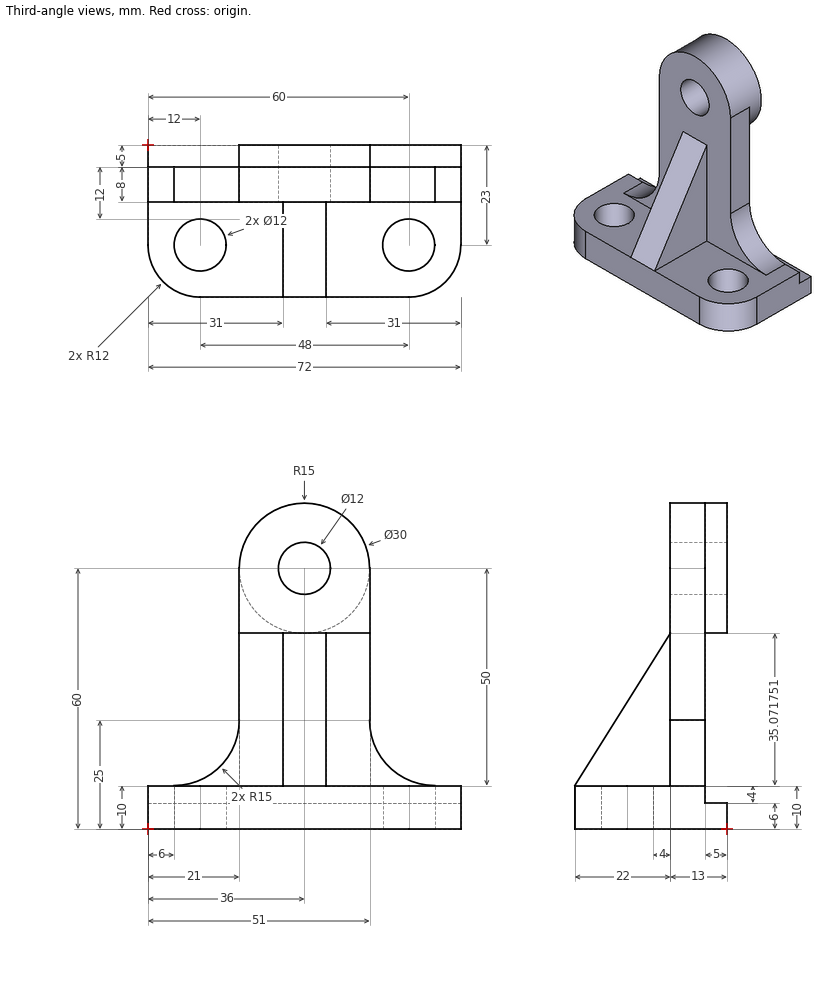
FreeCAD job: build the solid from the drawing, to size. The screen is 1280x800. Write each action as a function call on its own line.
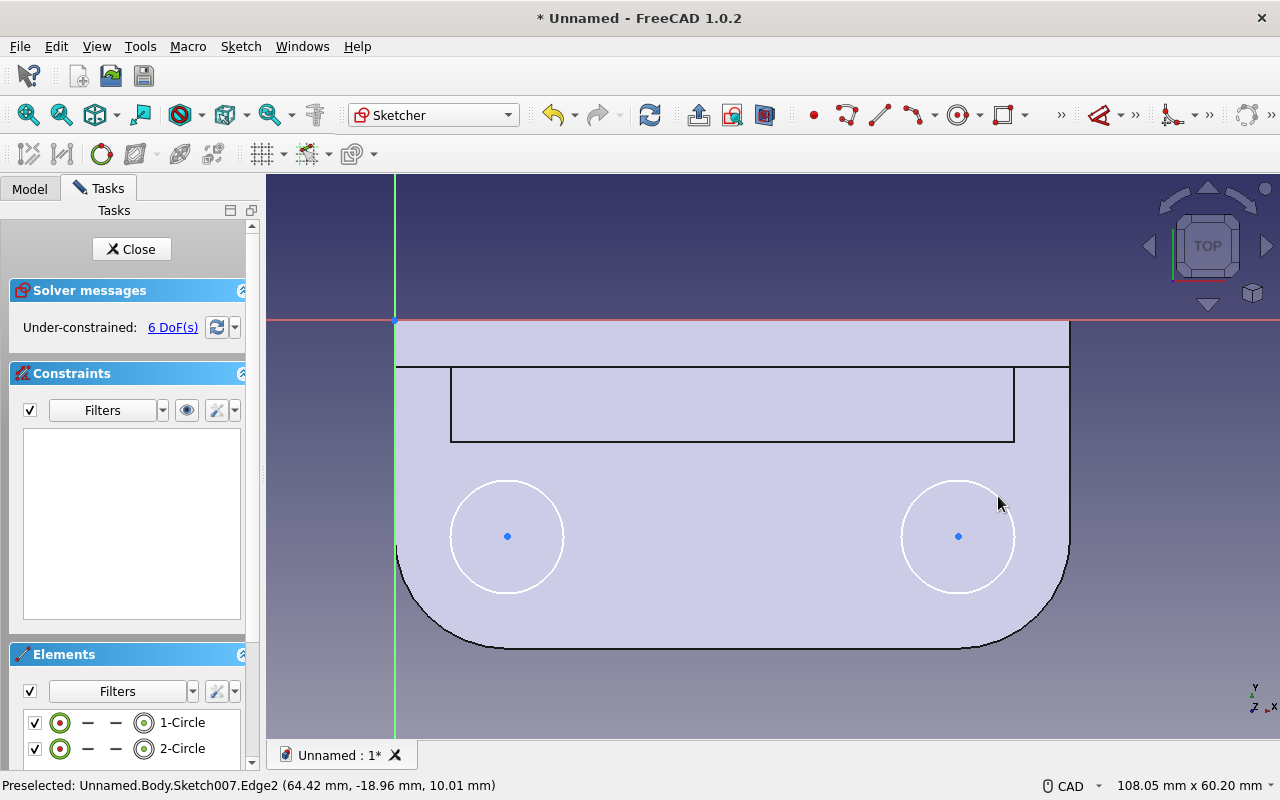
click(547, 497)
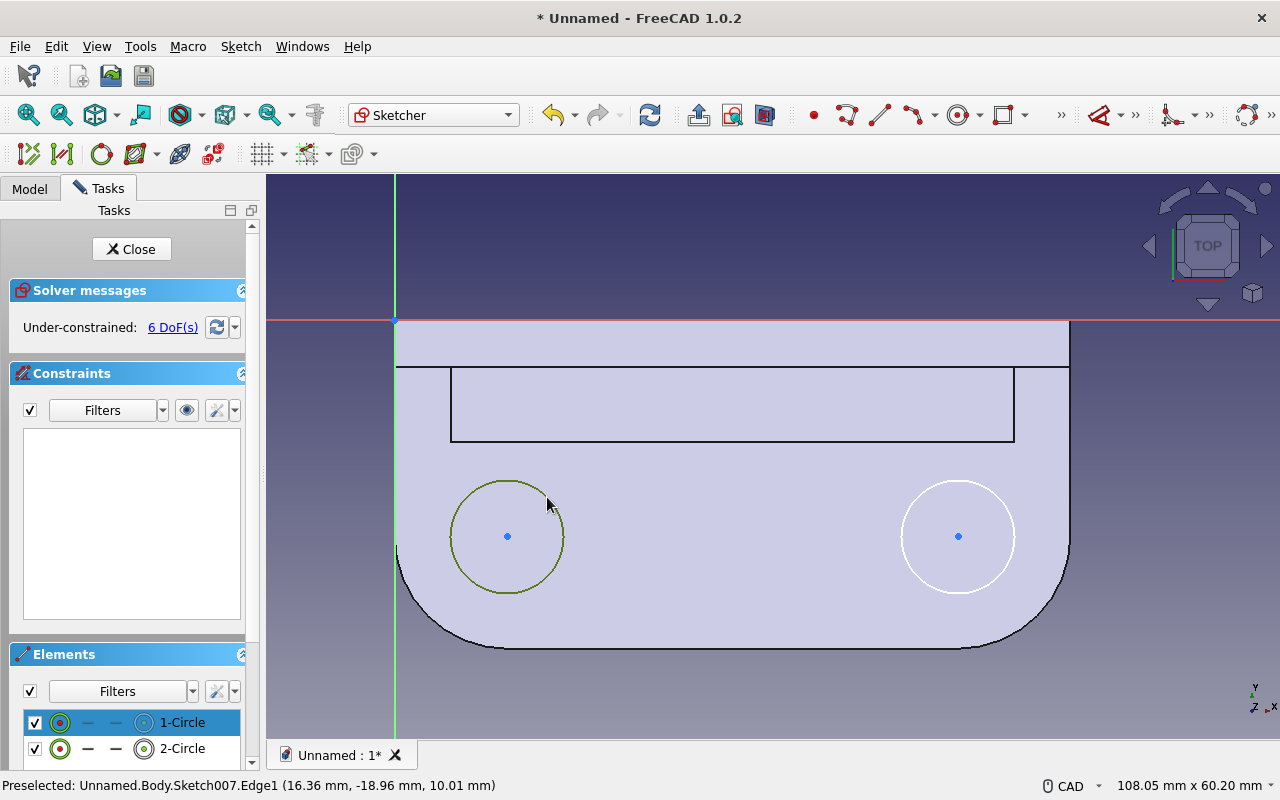
click(998, 497)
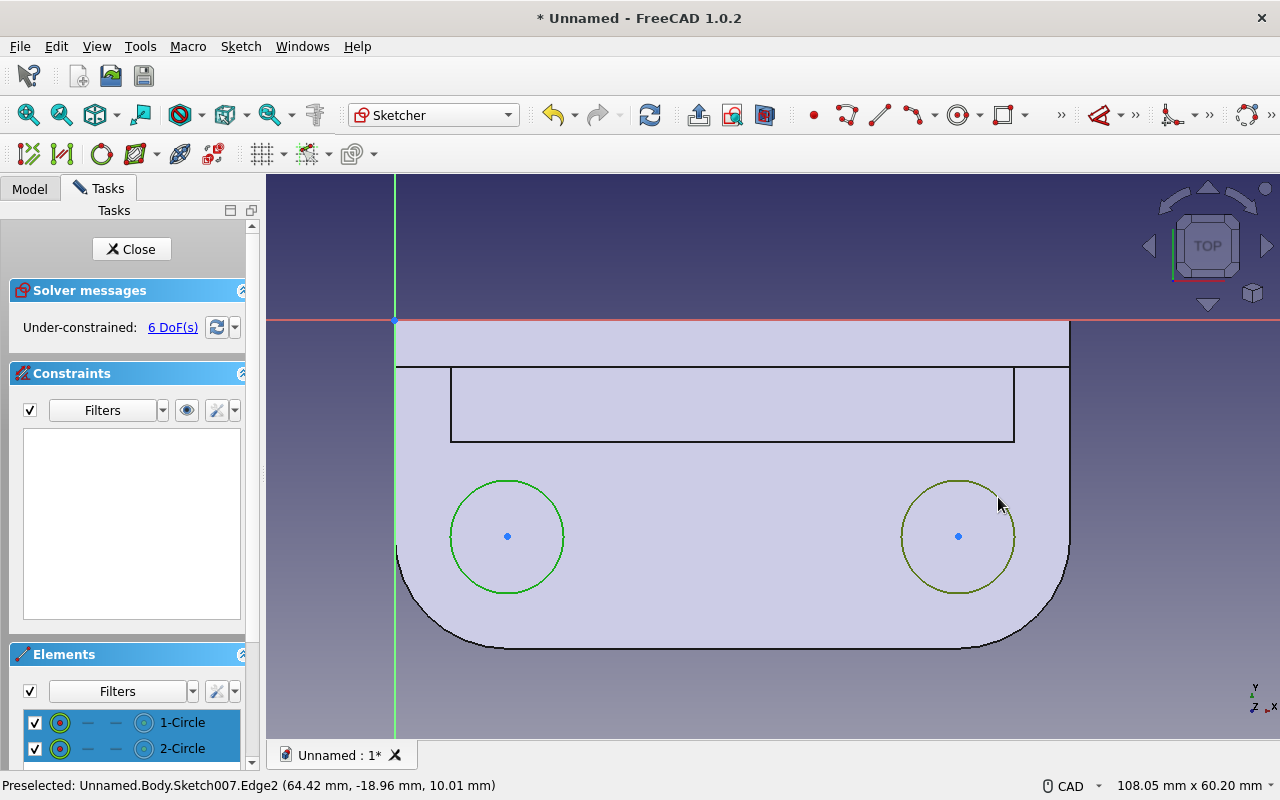
key(e)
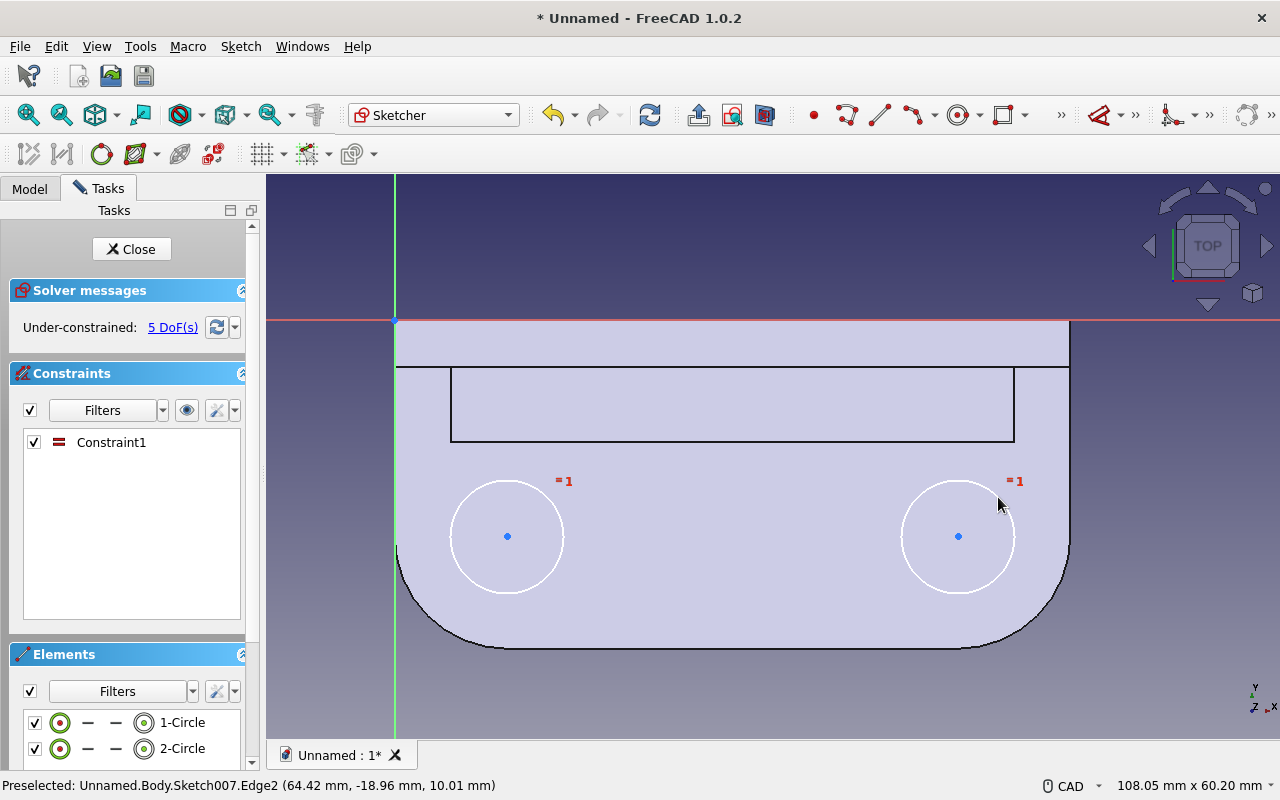
click(507, 537)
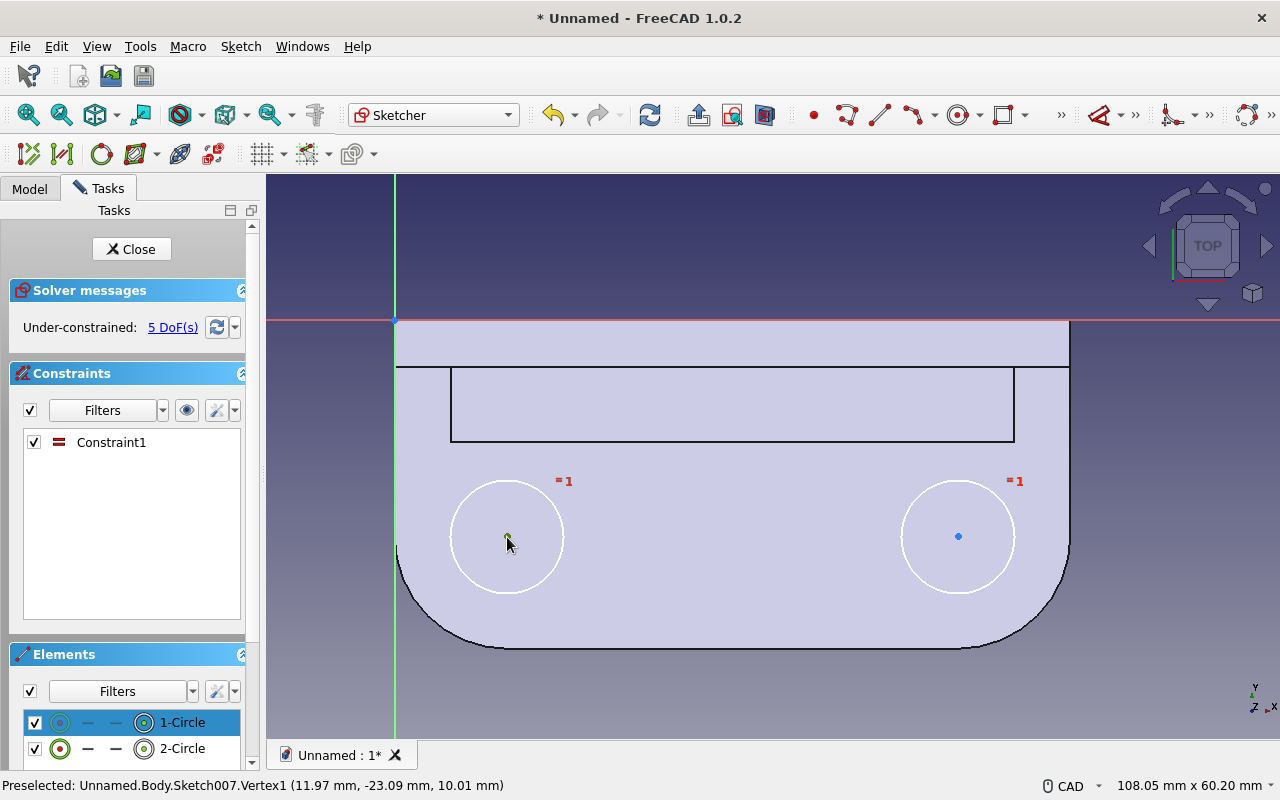
click(958, 537)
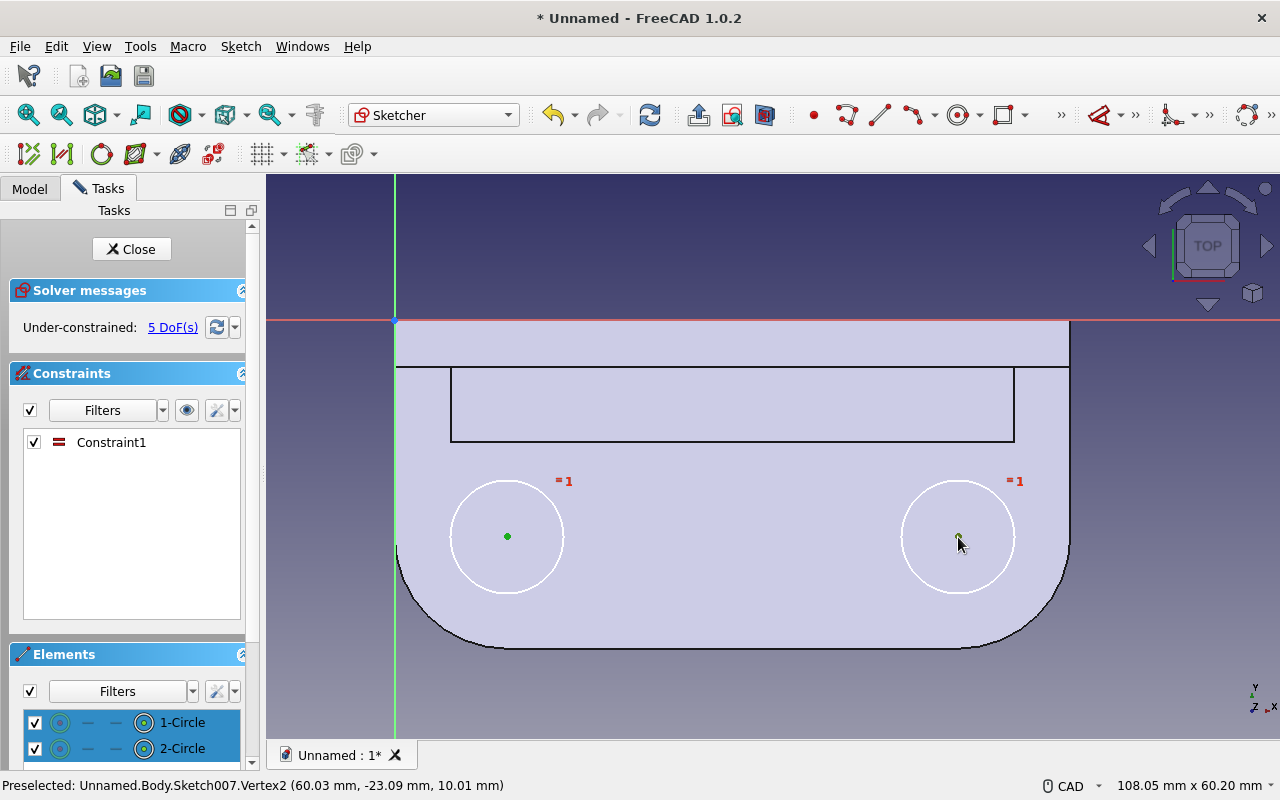
key(h)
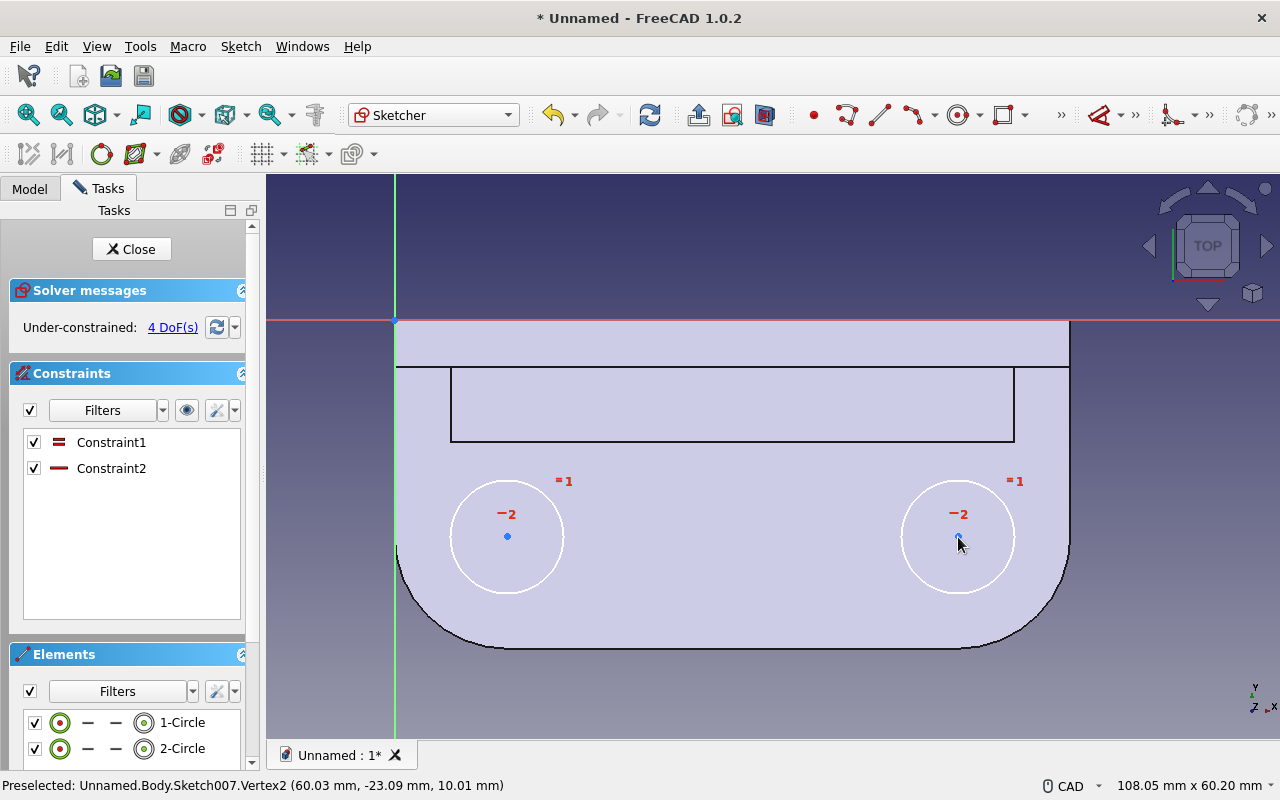
click(1098, 116)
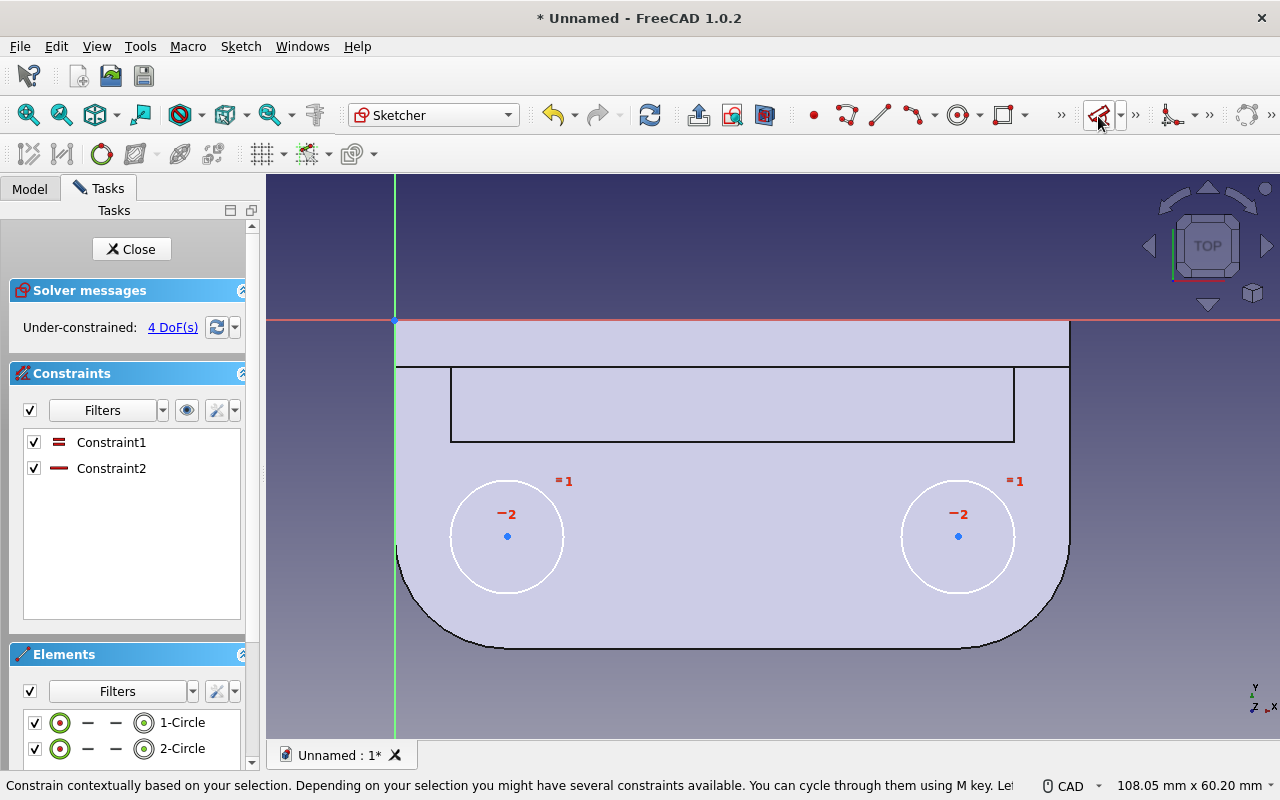
click(547, 497)
click(570, 474)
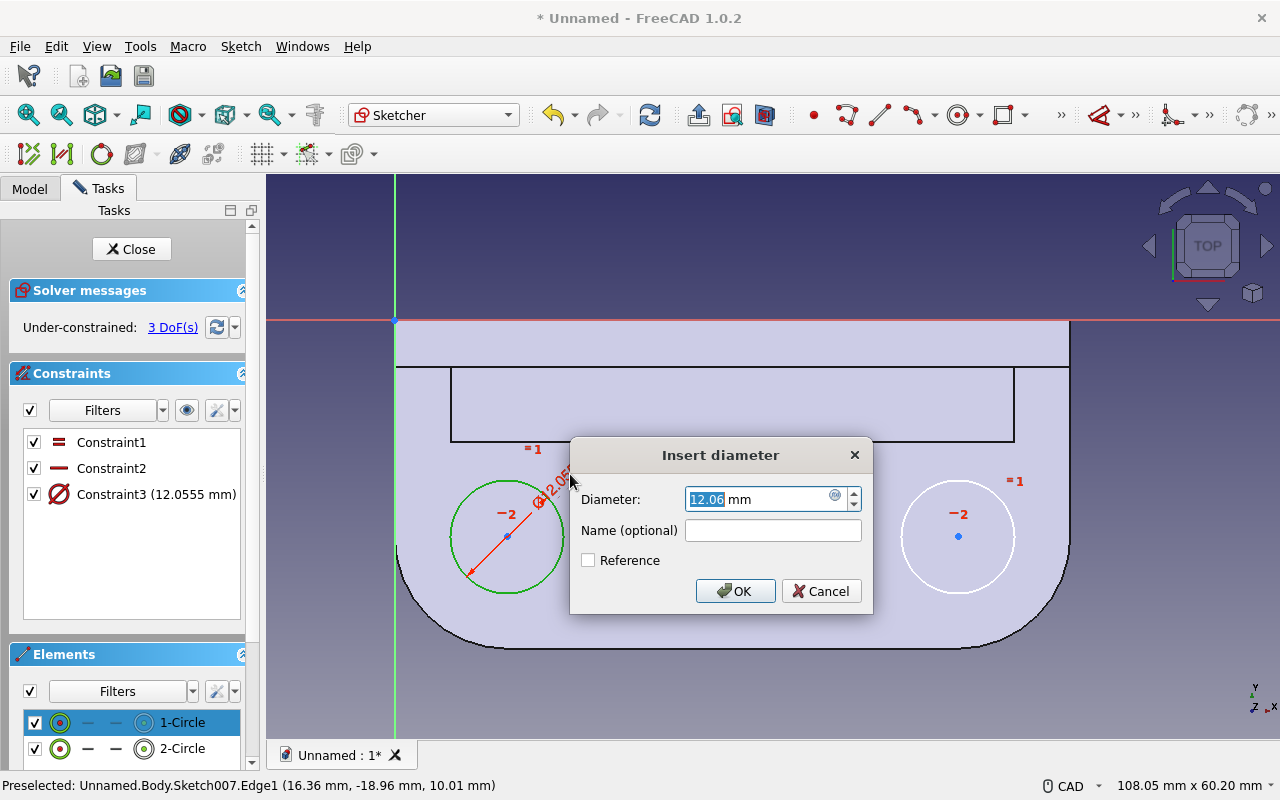
text(12)
key(Return)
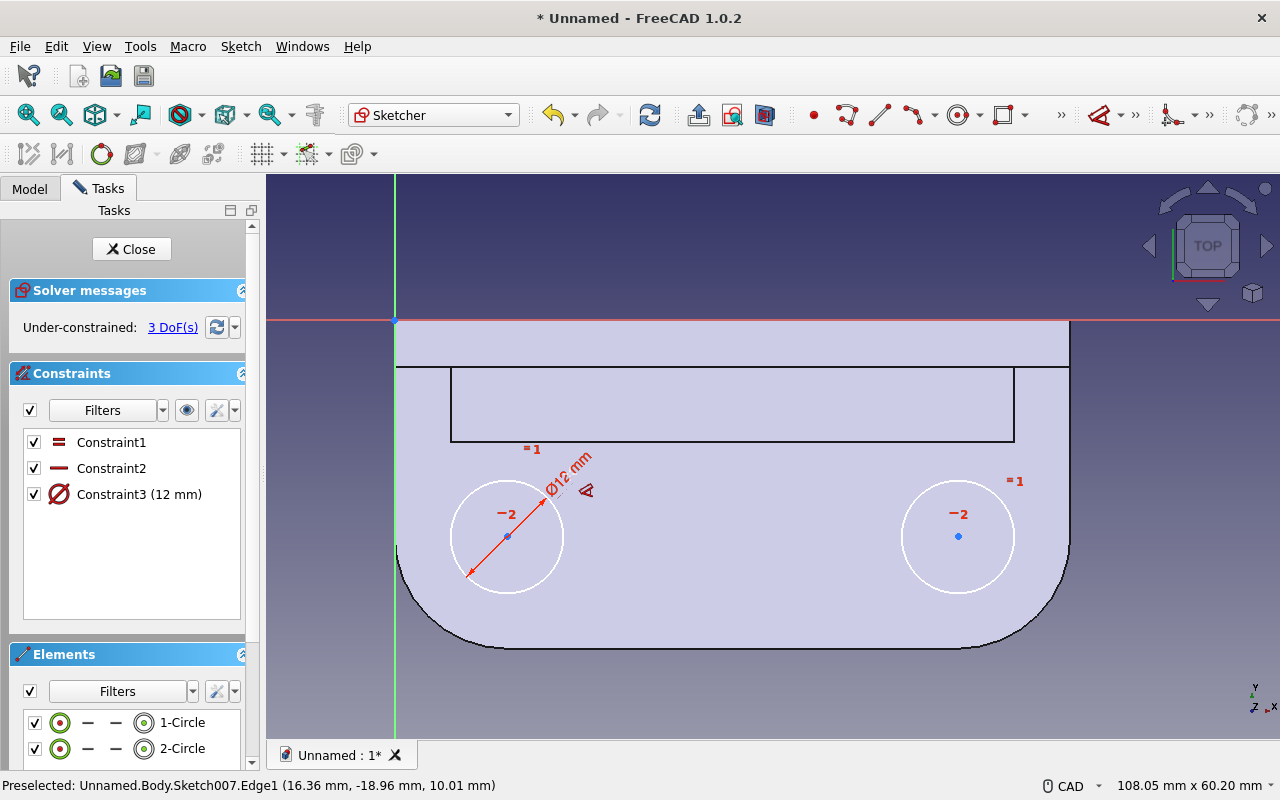
click(507, 537)
click(451, 286)